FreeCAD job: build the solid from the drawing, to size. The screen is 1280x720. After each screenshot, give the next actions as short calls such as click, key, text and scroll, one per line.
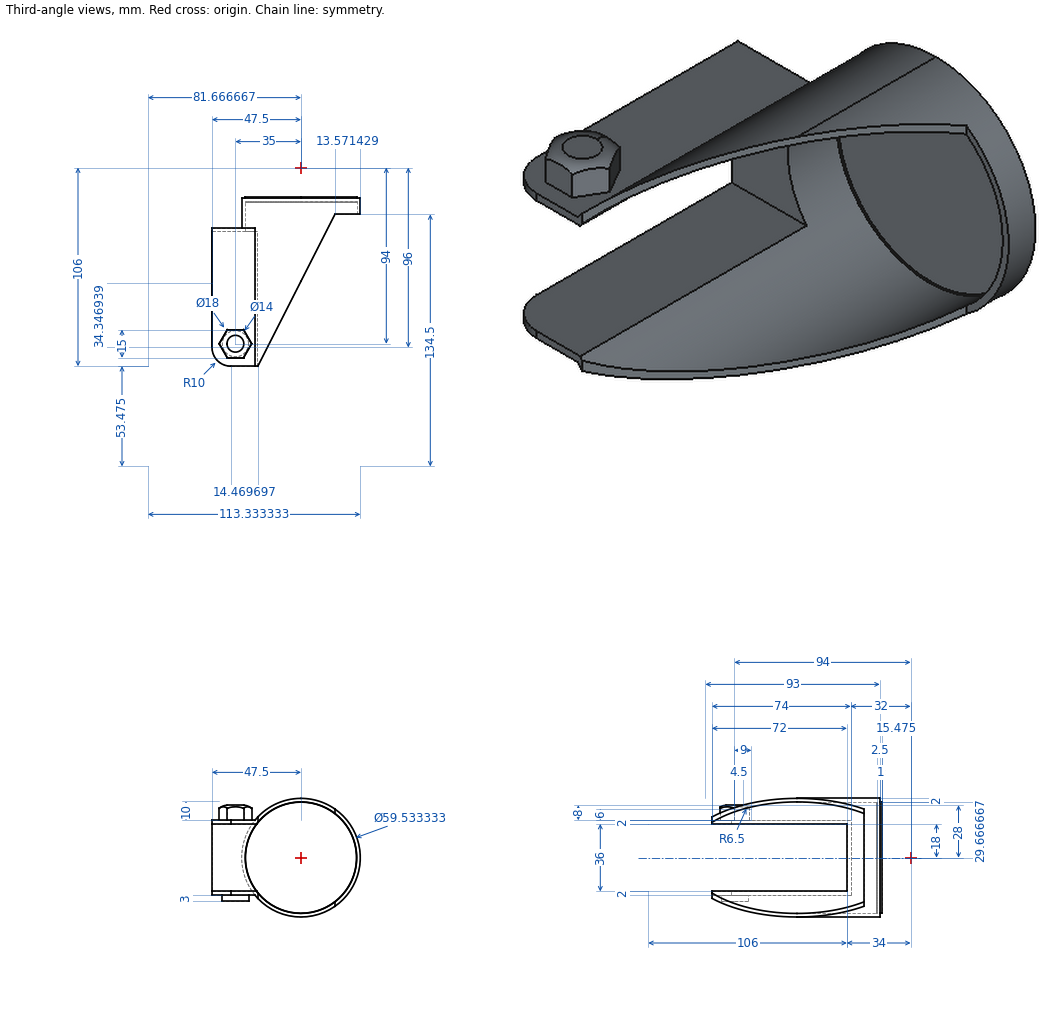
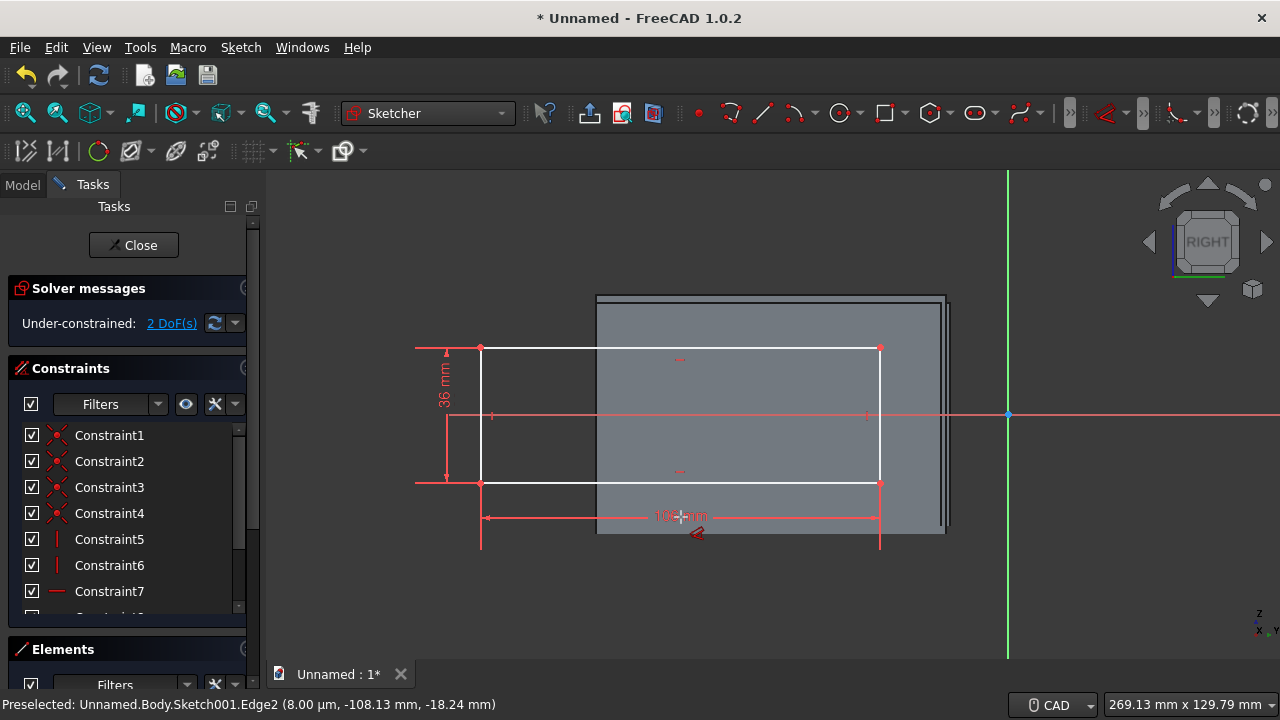
click(481, 348)
click(447, 358)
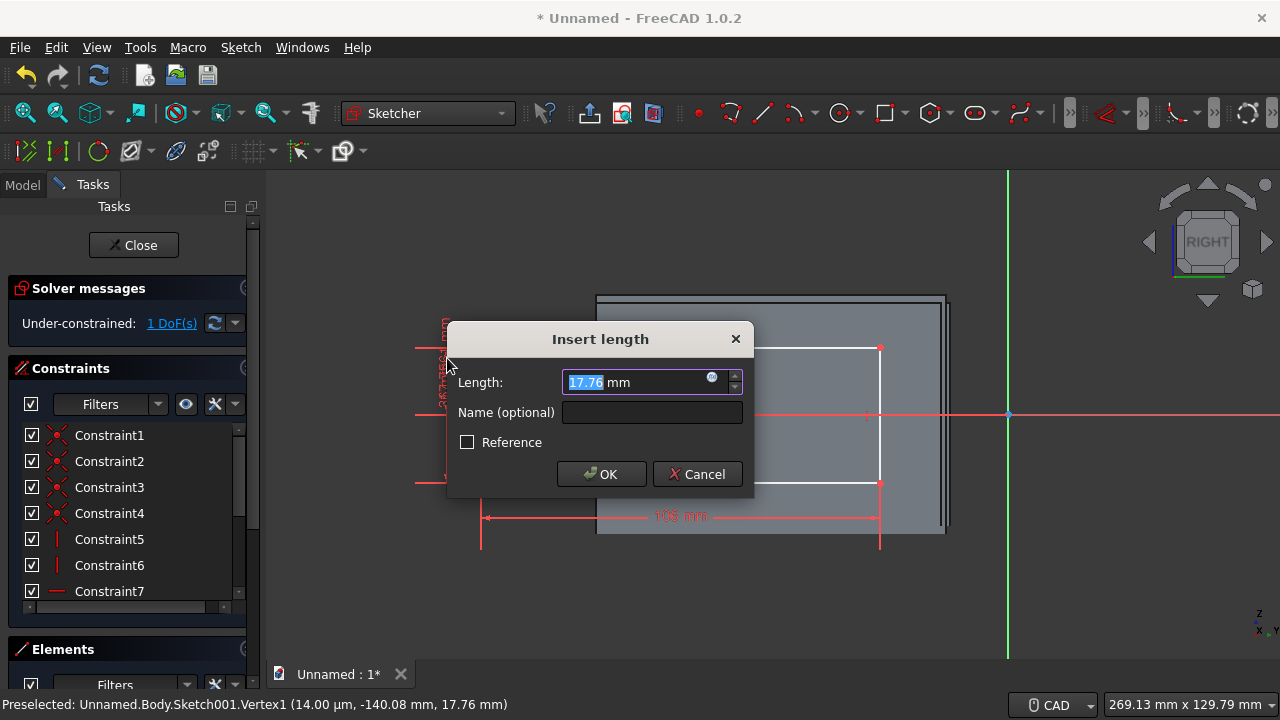
text(18)
key(Return)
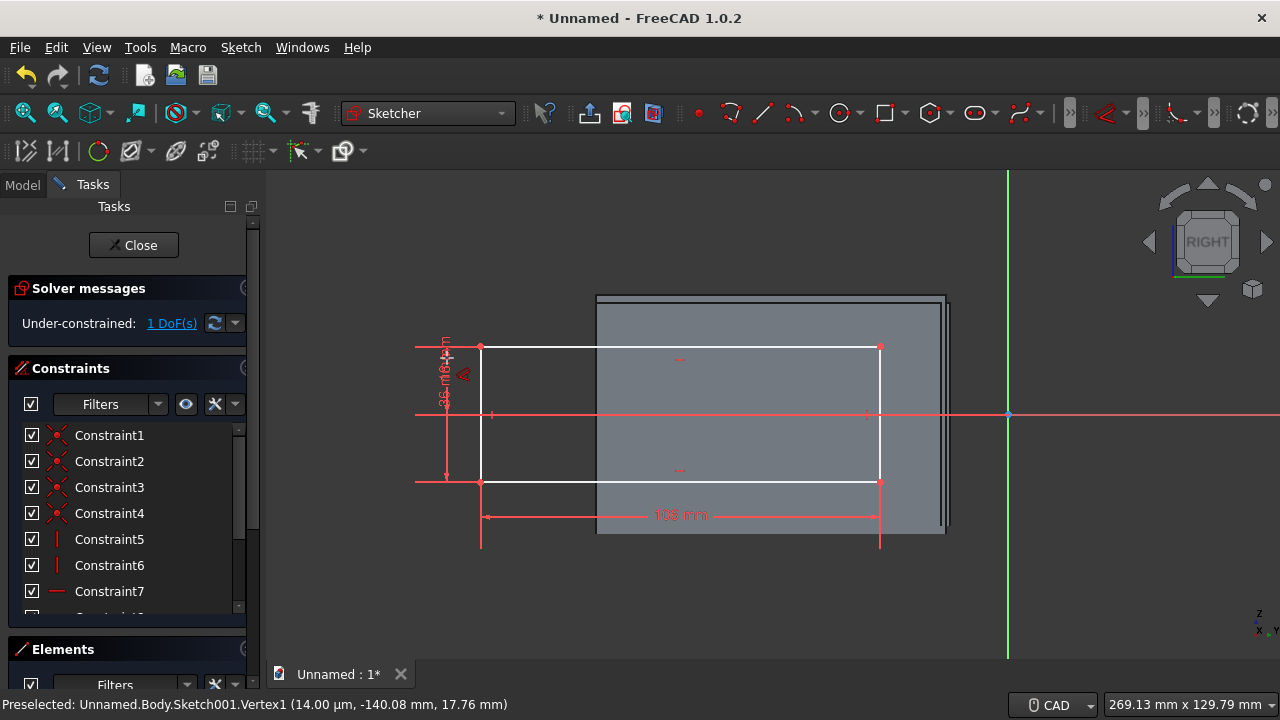
click(880, 482)
click(944, 516)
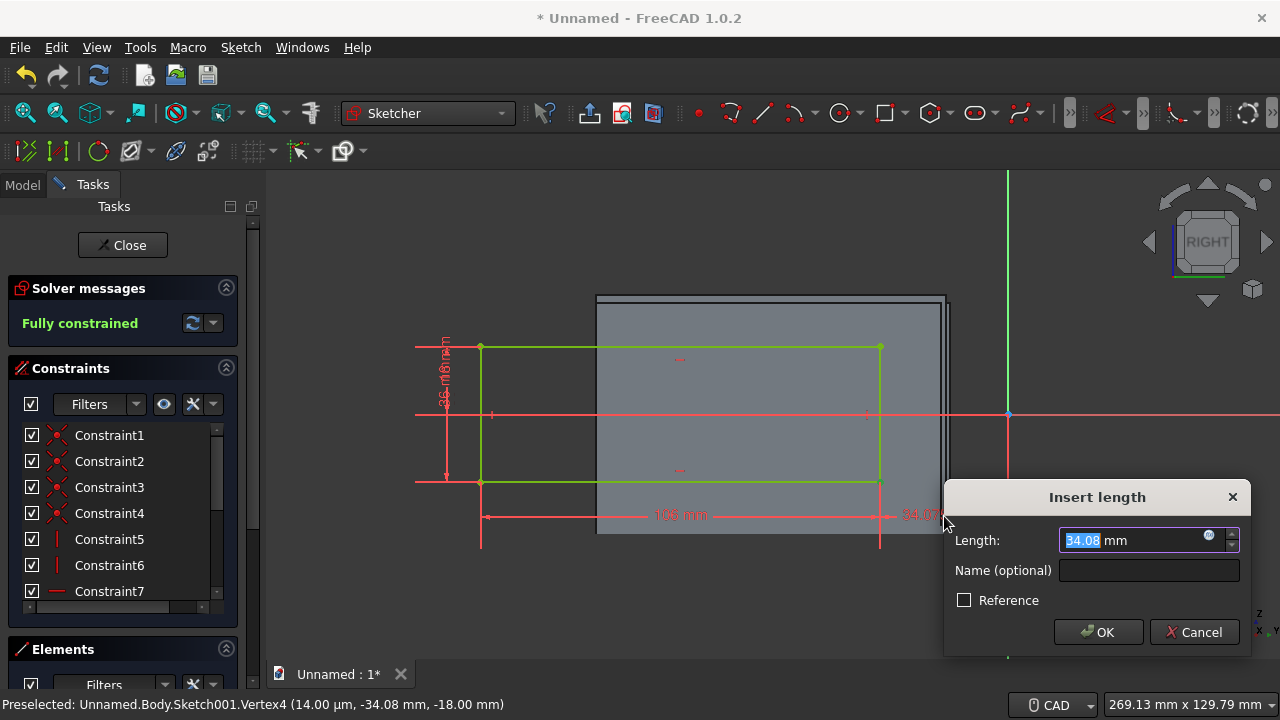
text(34)
key(Return)
key(Escape)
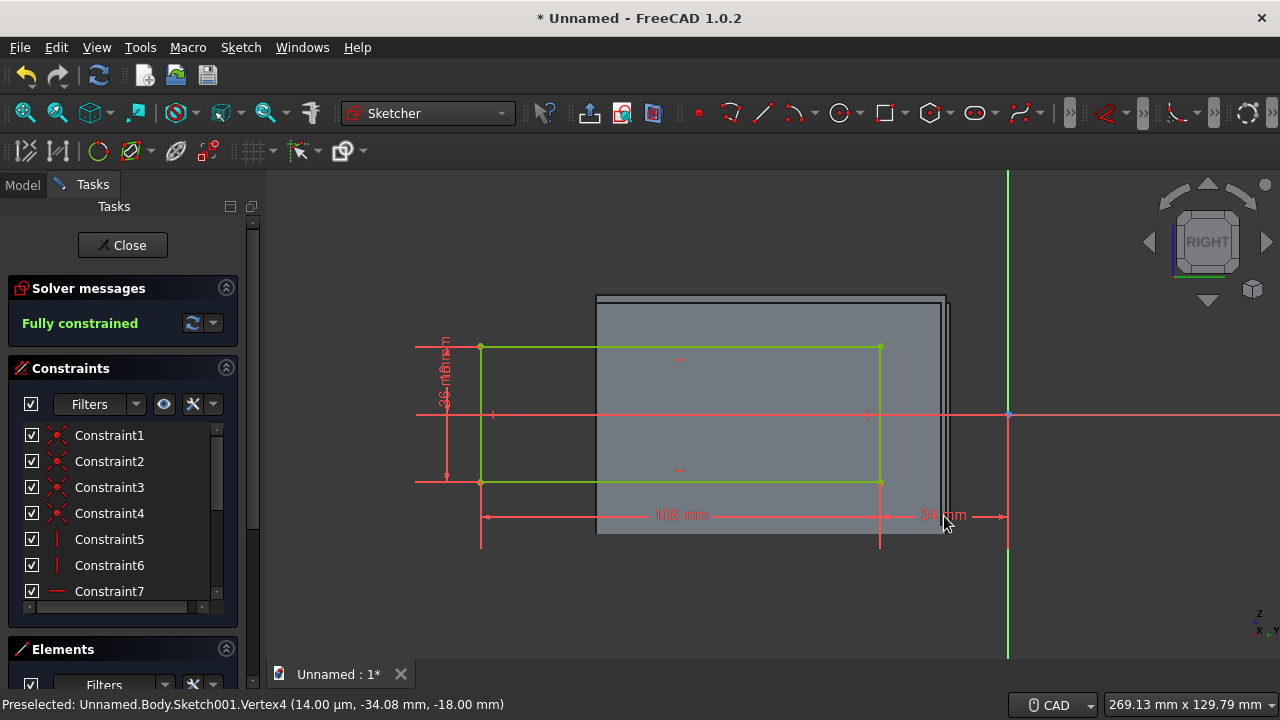
click(123, 245)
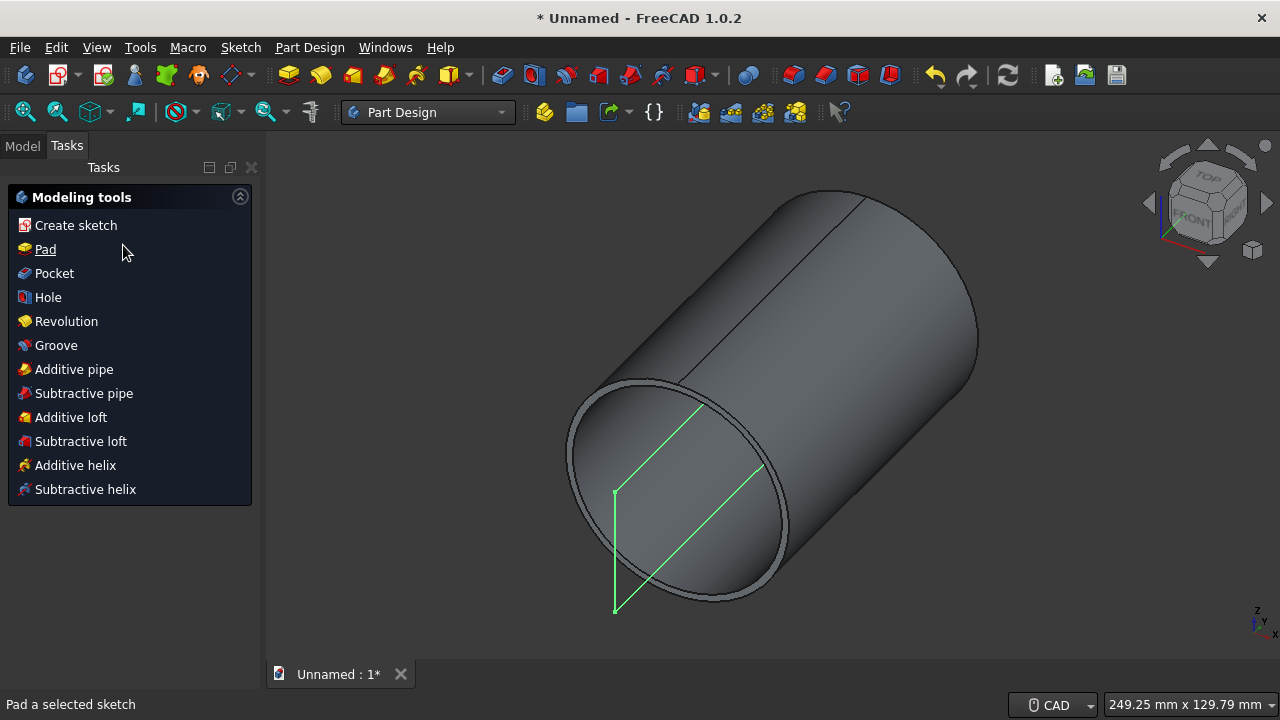
click(504, 76)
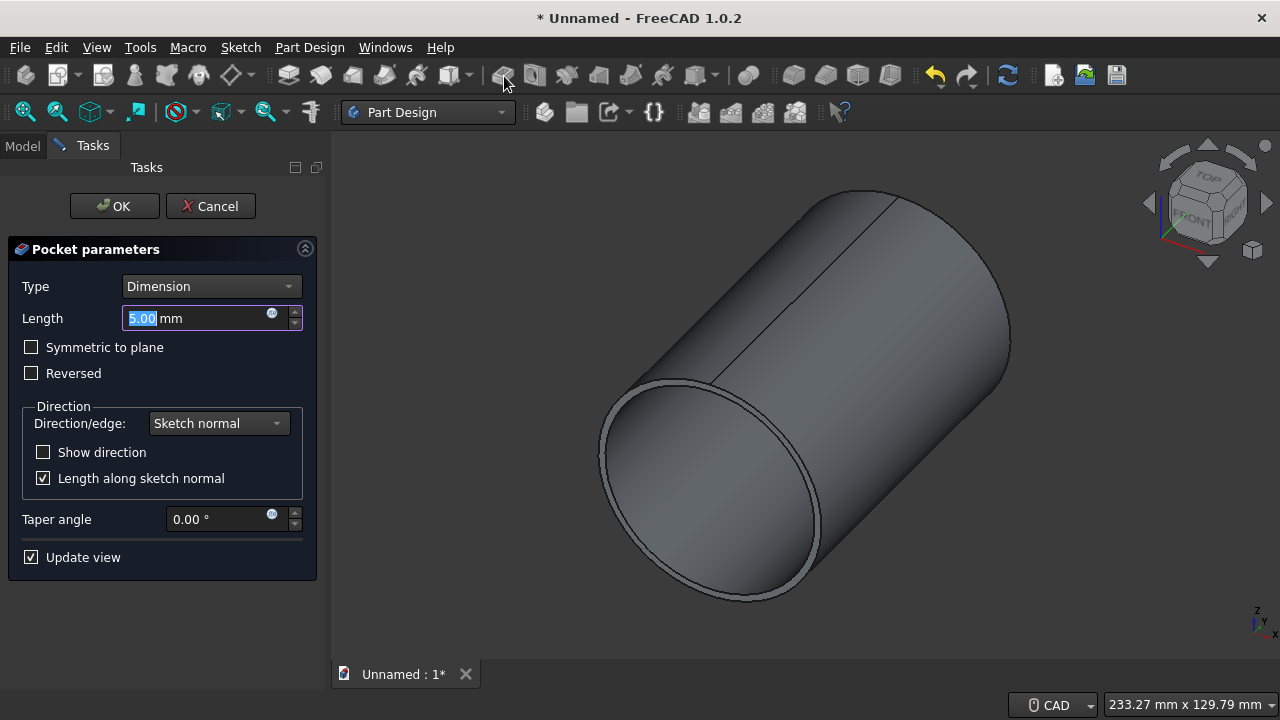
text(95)
key(Tab)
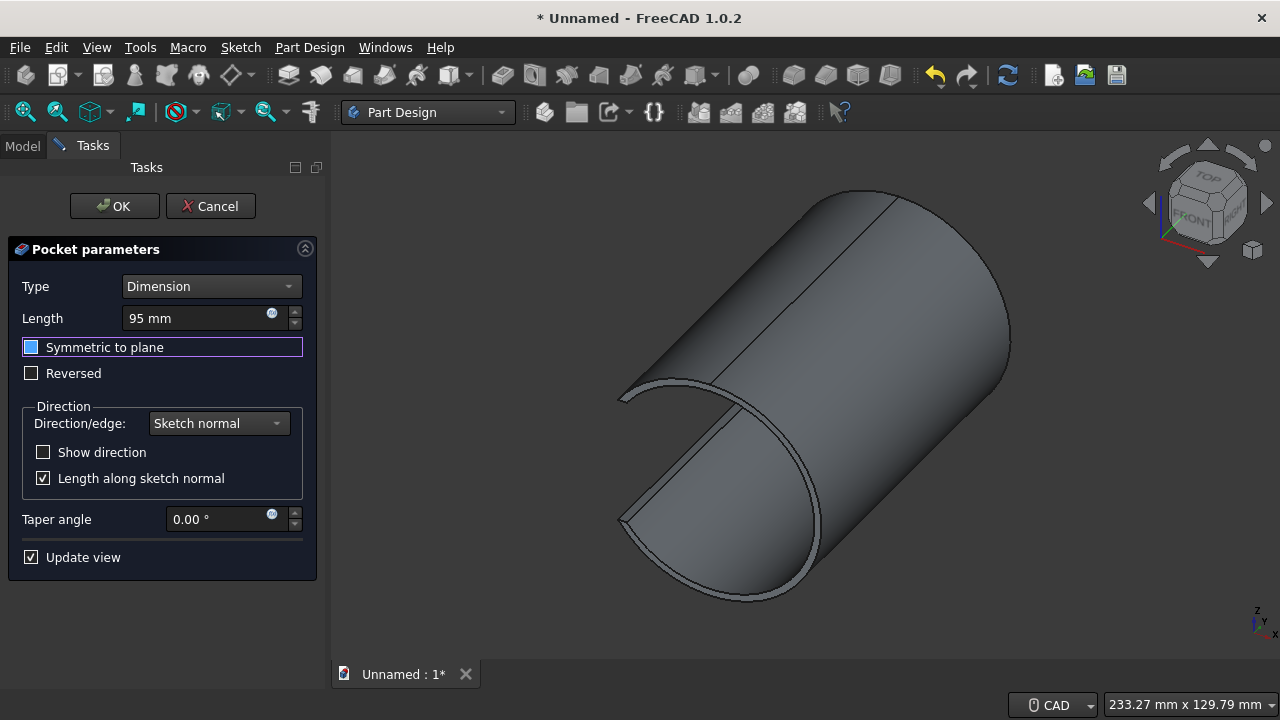
click(115, 206)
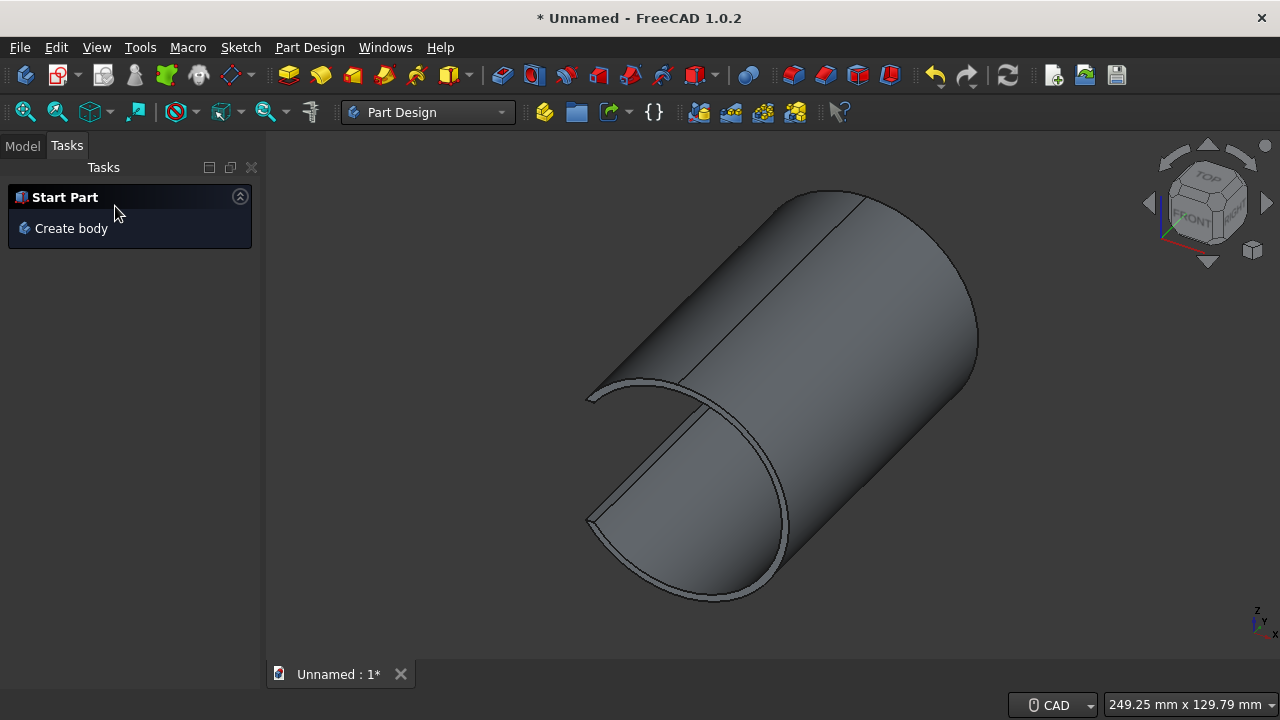
click(58, 76)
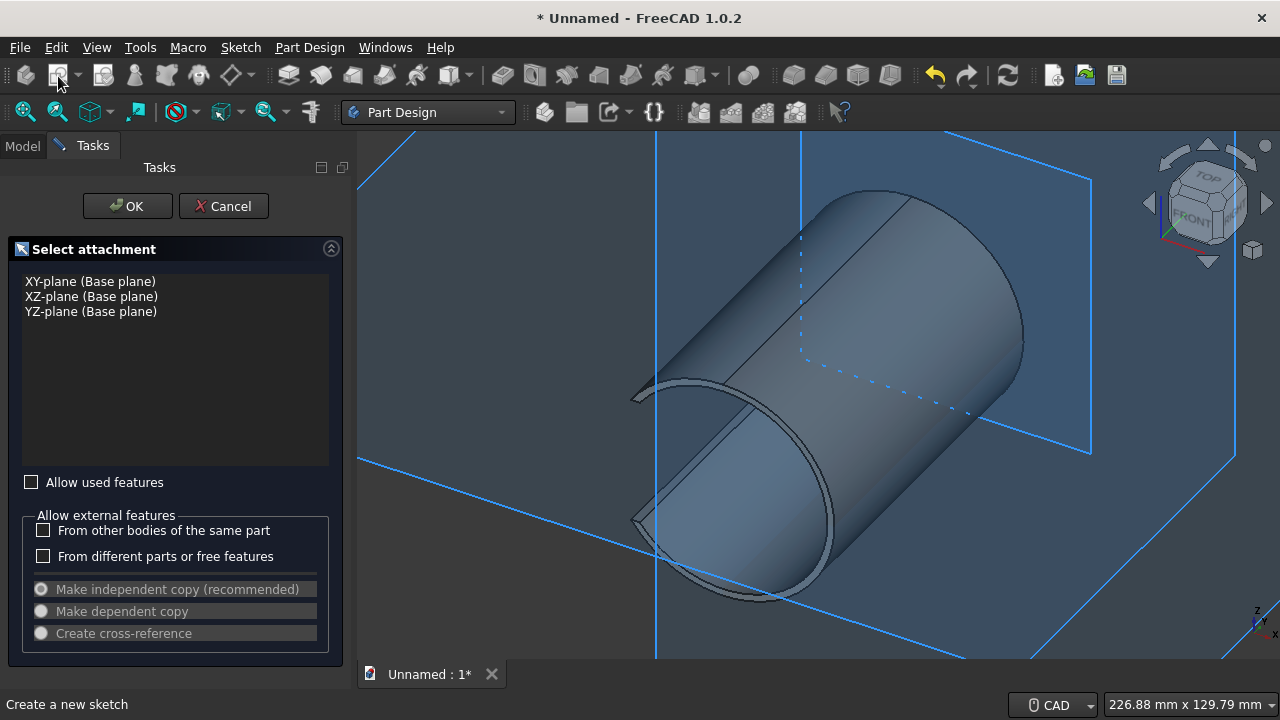
click(82, 312)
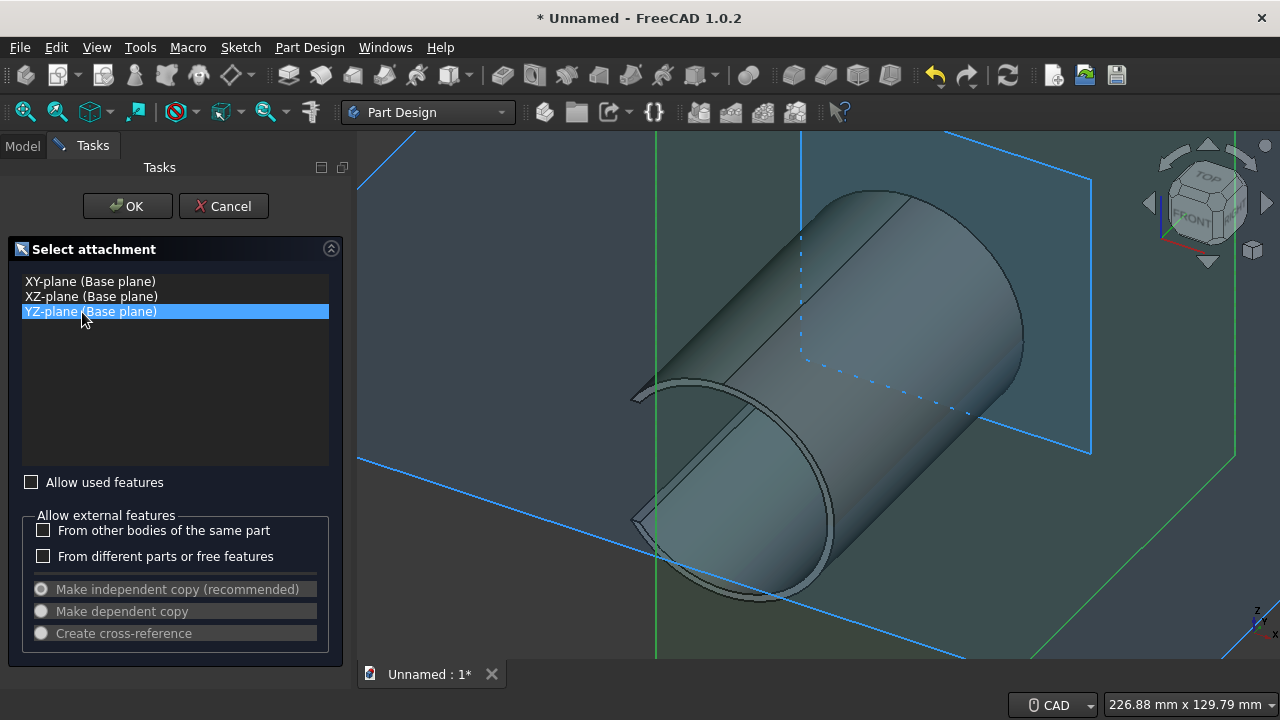
click(128, 206)